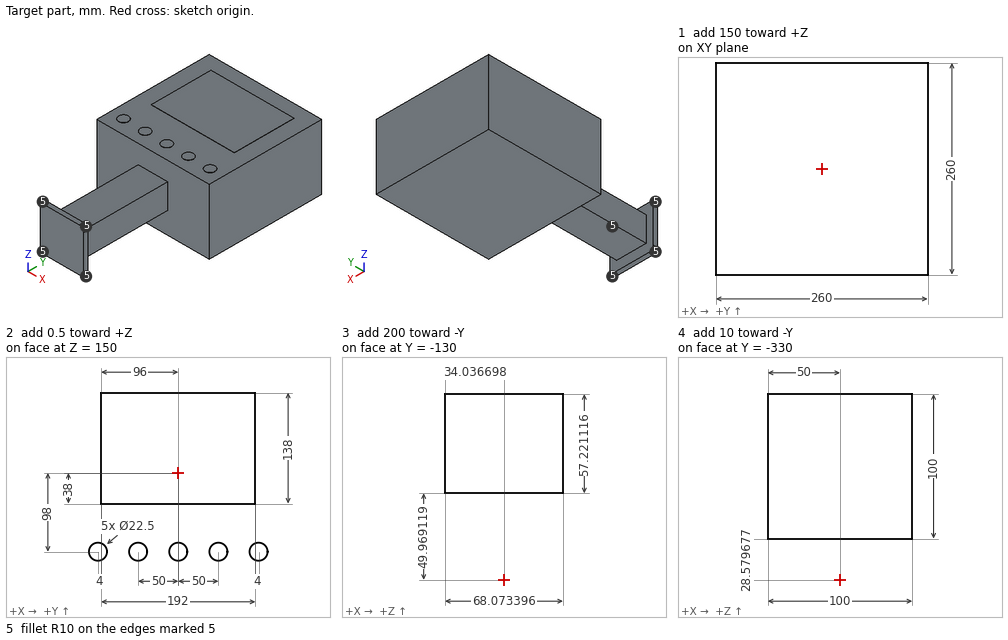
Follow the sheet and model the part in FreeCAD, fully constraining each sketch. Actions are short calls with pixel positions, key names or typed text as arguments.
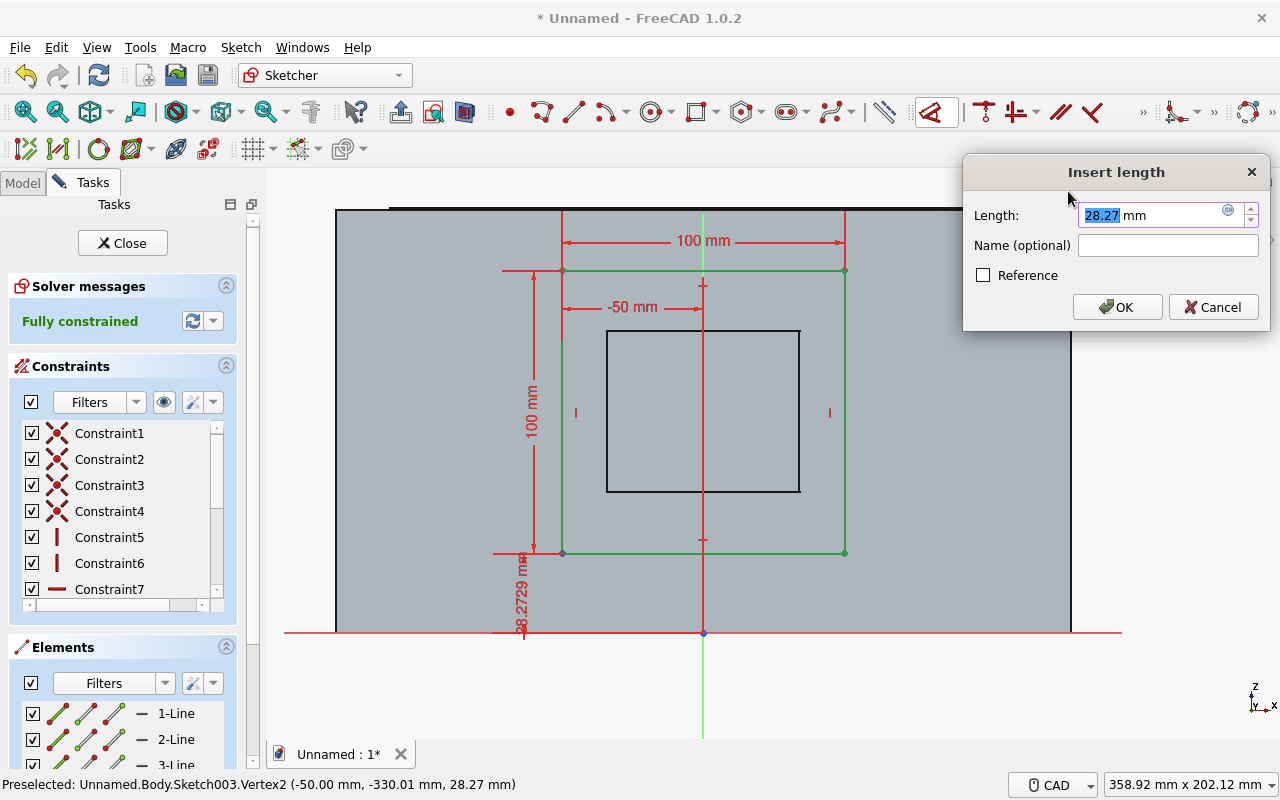
text(28.579677)
key(Return)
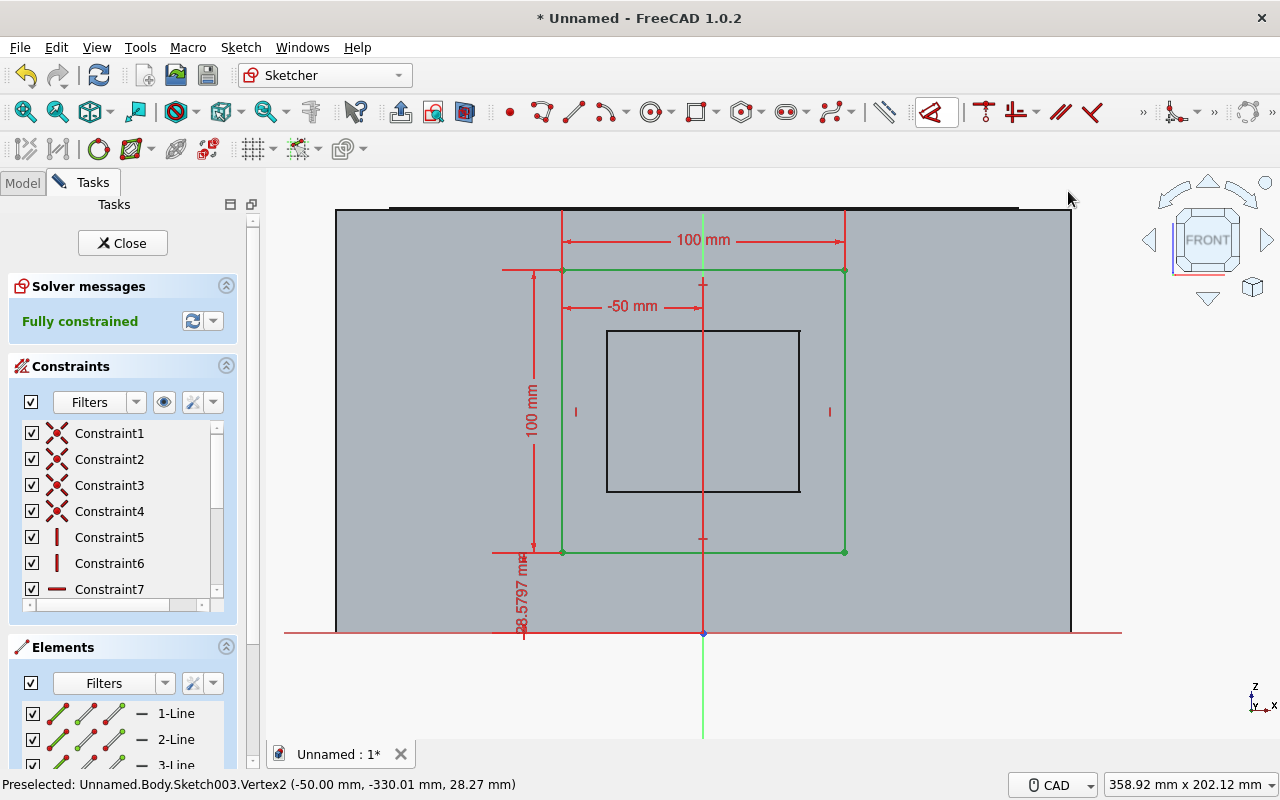
click(123, 243)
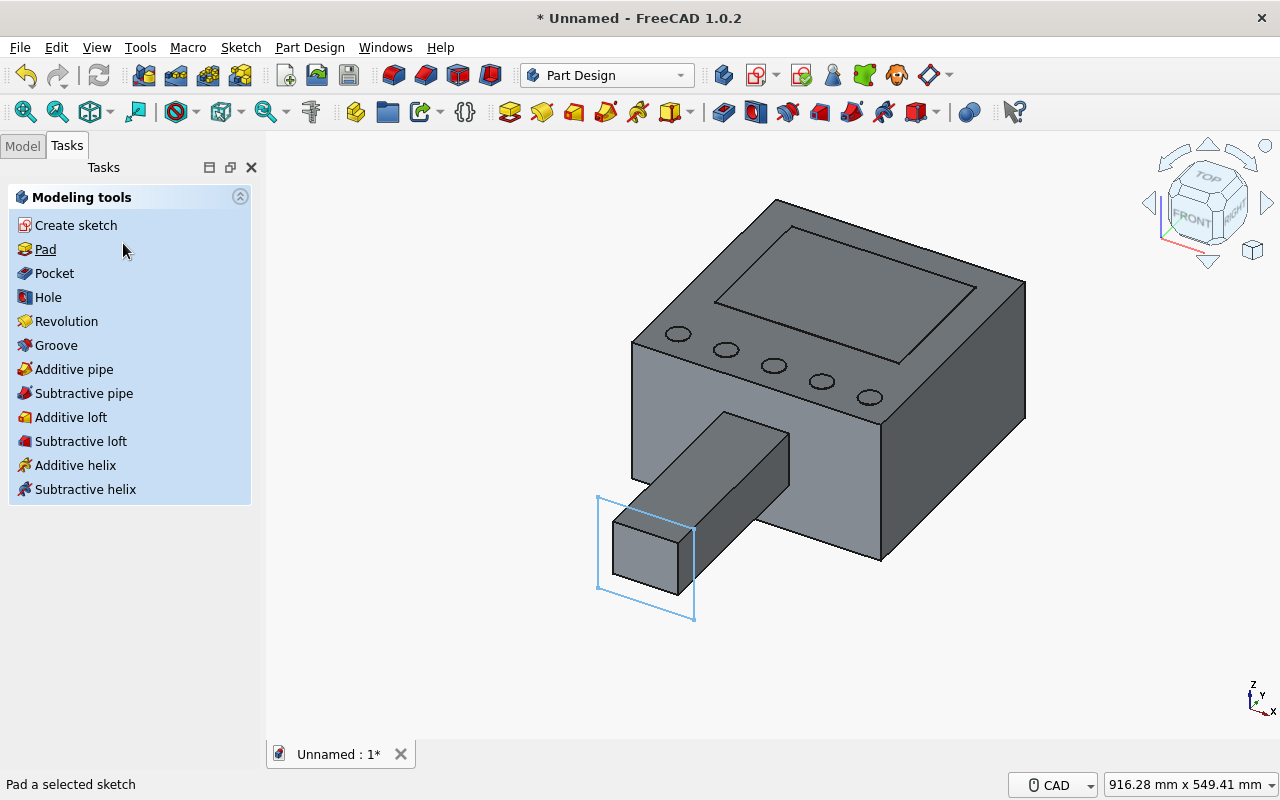
click(510, 112)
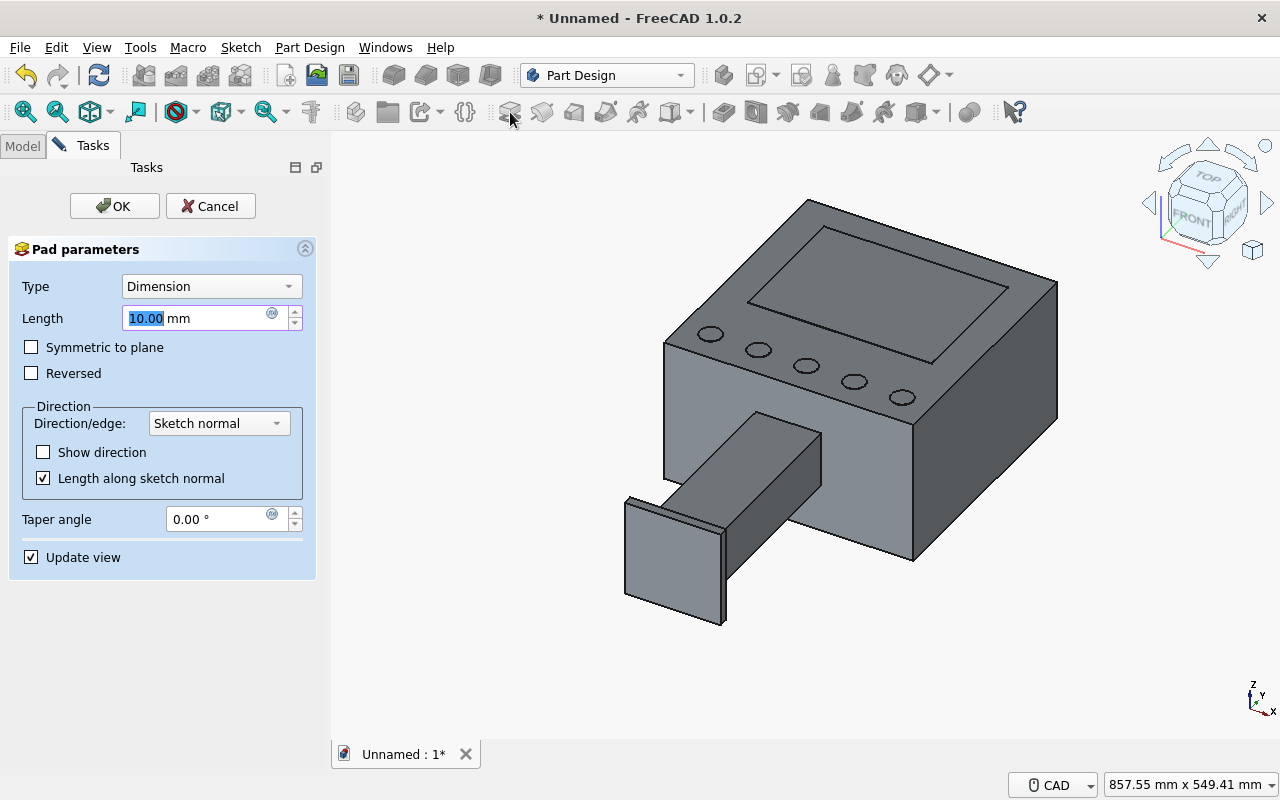
text(10)
key(Tab)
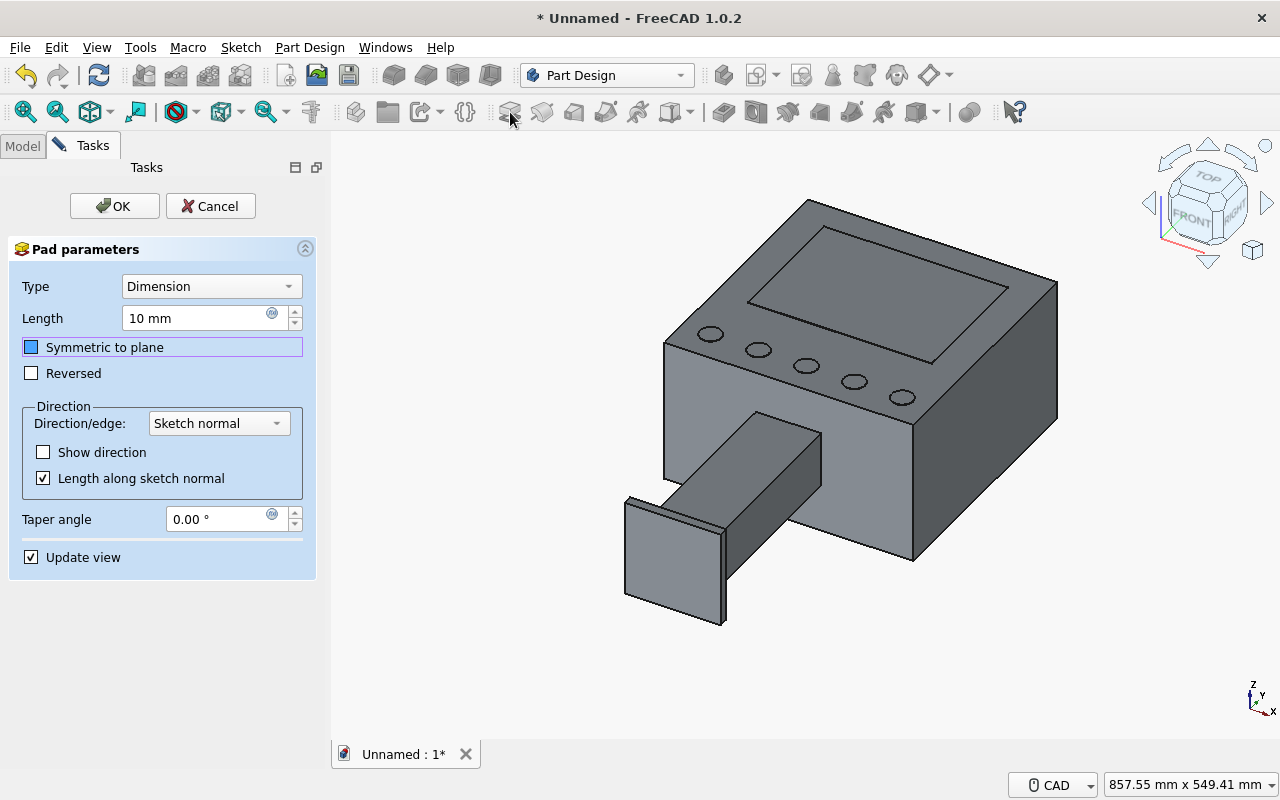
click(115, 206)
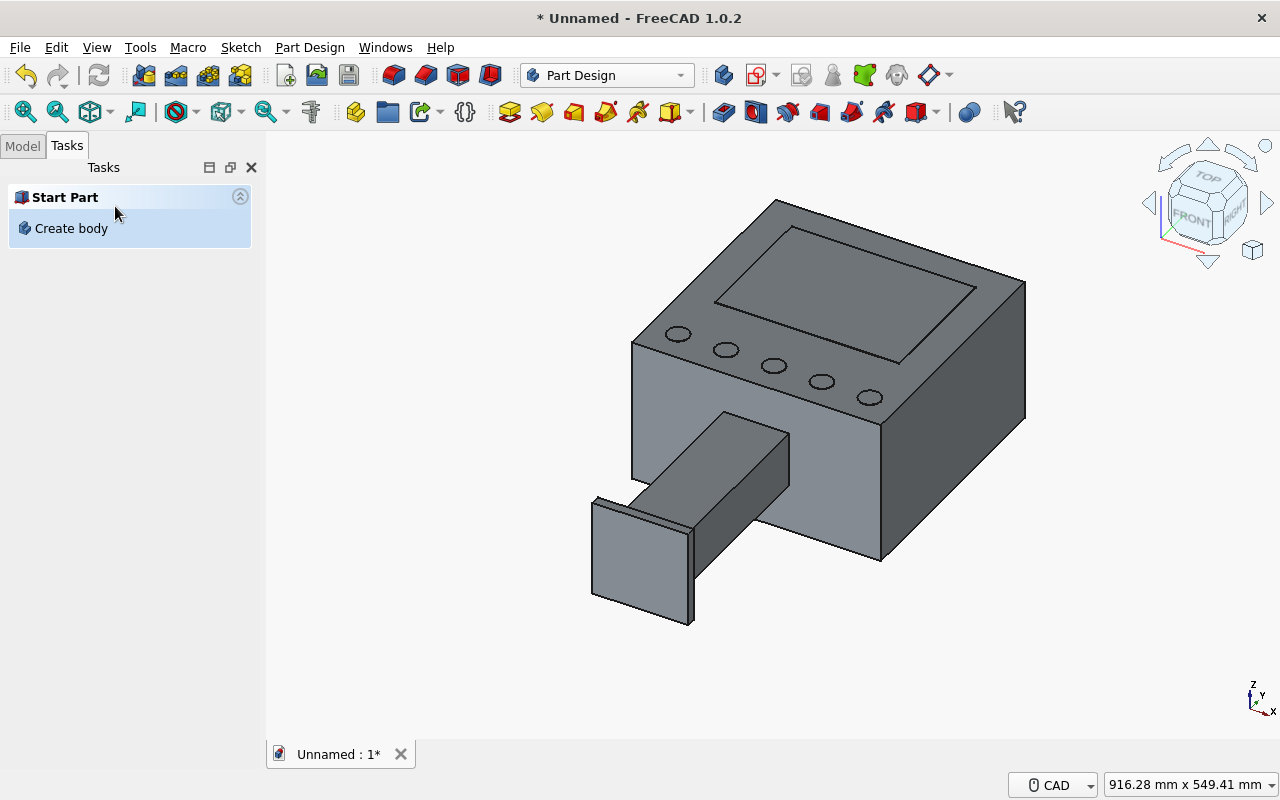
scroll(691, 621, up, 7)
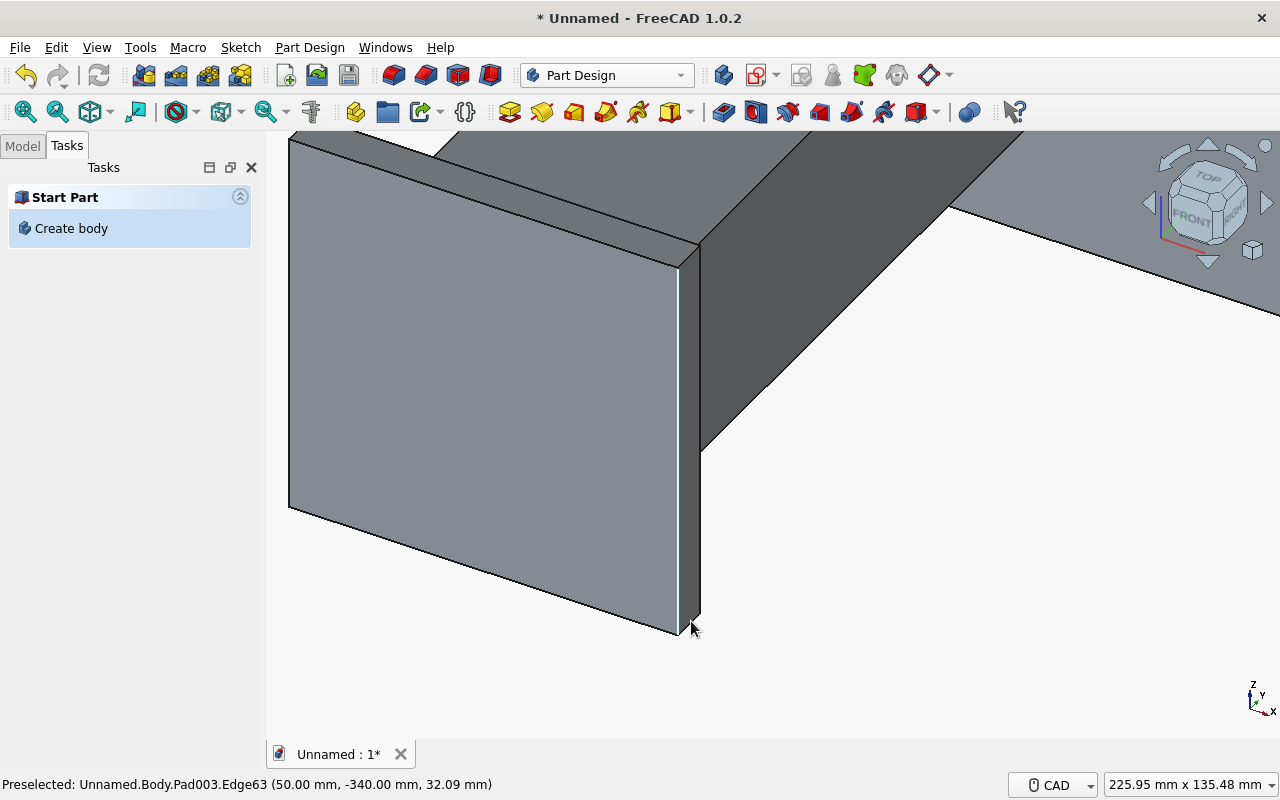
click(689, 256)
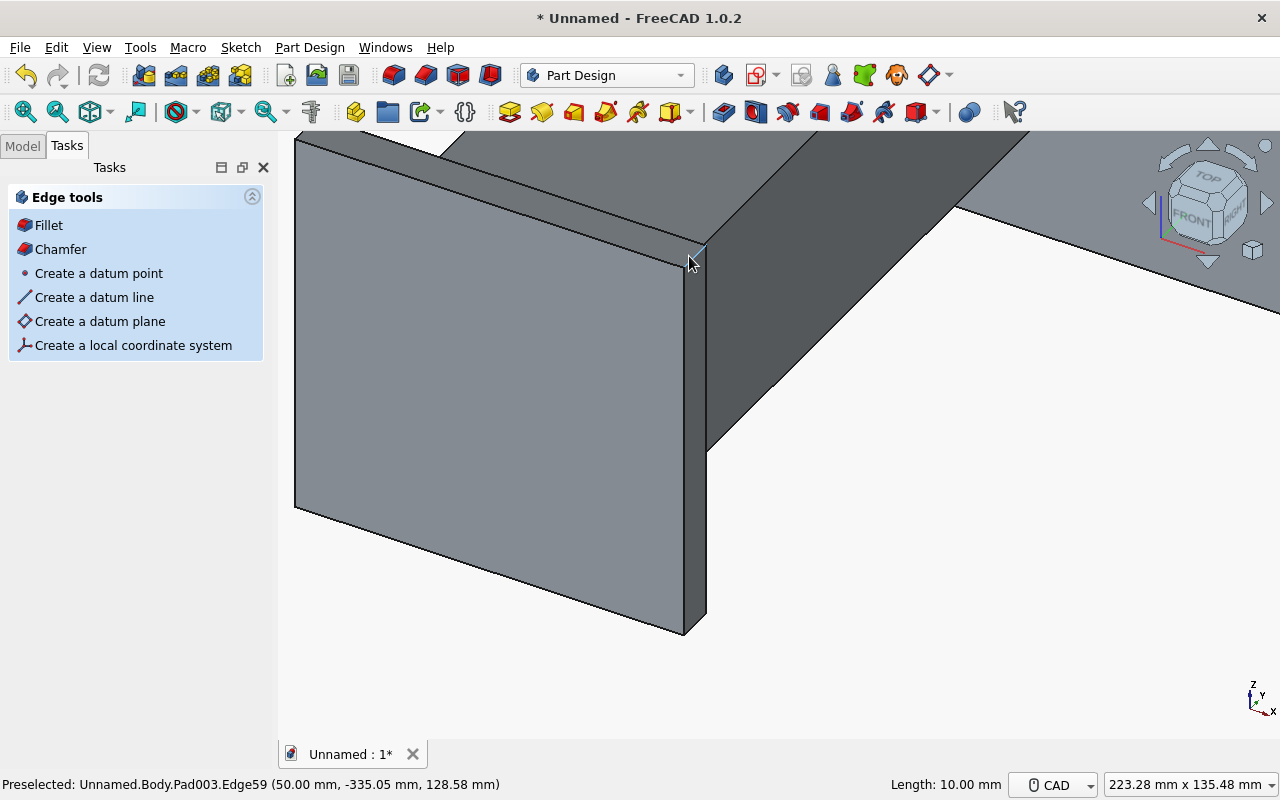
click(26, 112)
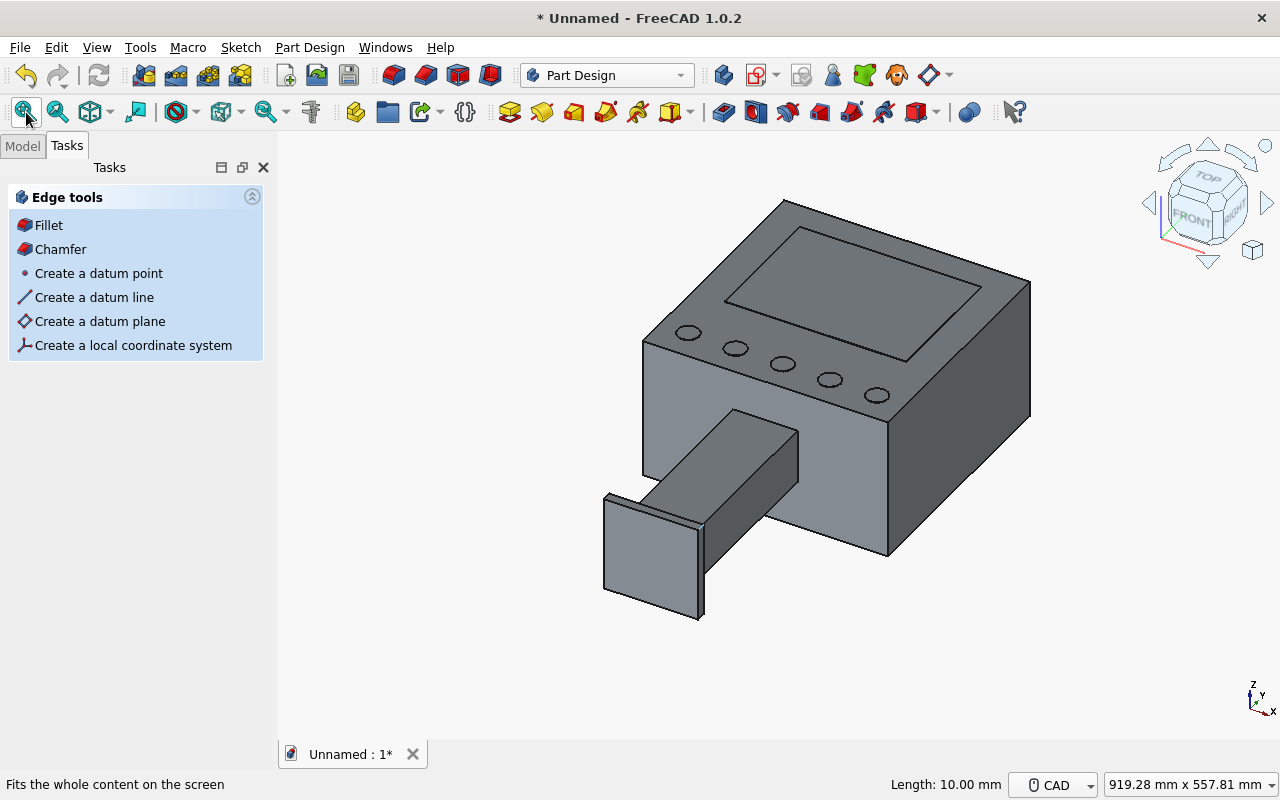
key(0)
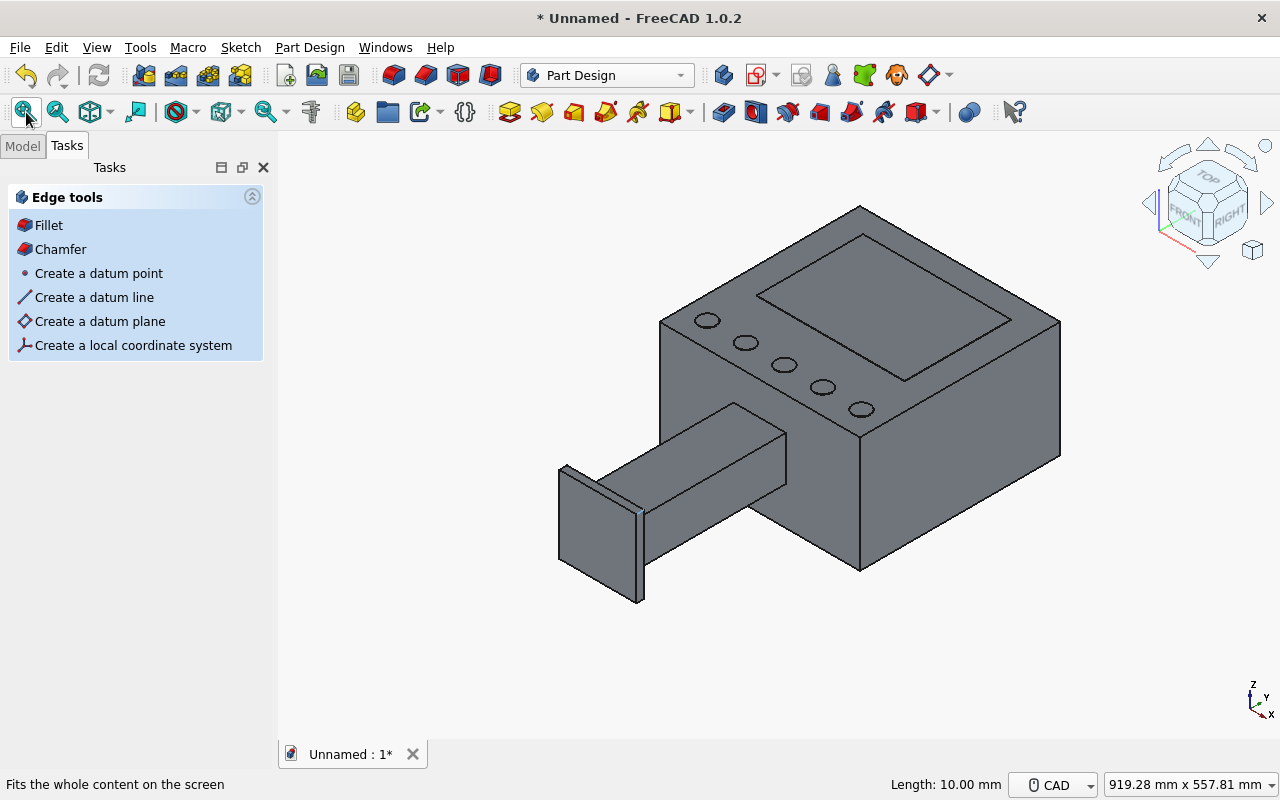
scroll(640, 600, up, 7)